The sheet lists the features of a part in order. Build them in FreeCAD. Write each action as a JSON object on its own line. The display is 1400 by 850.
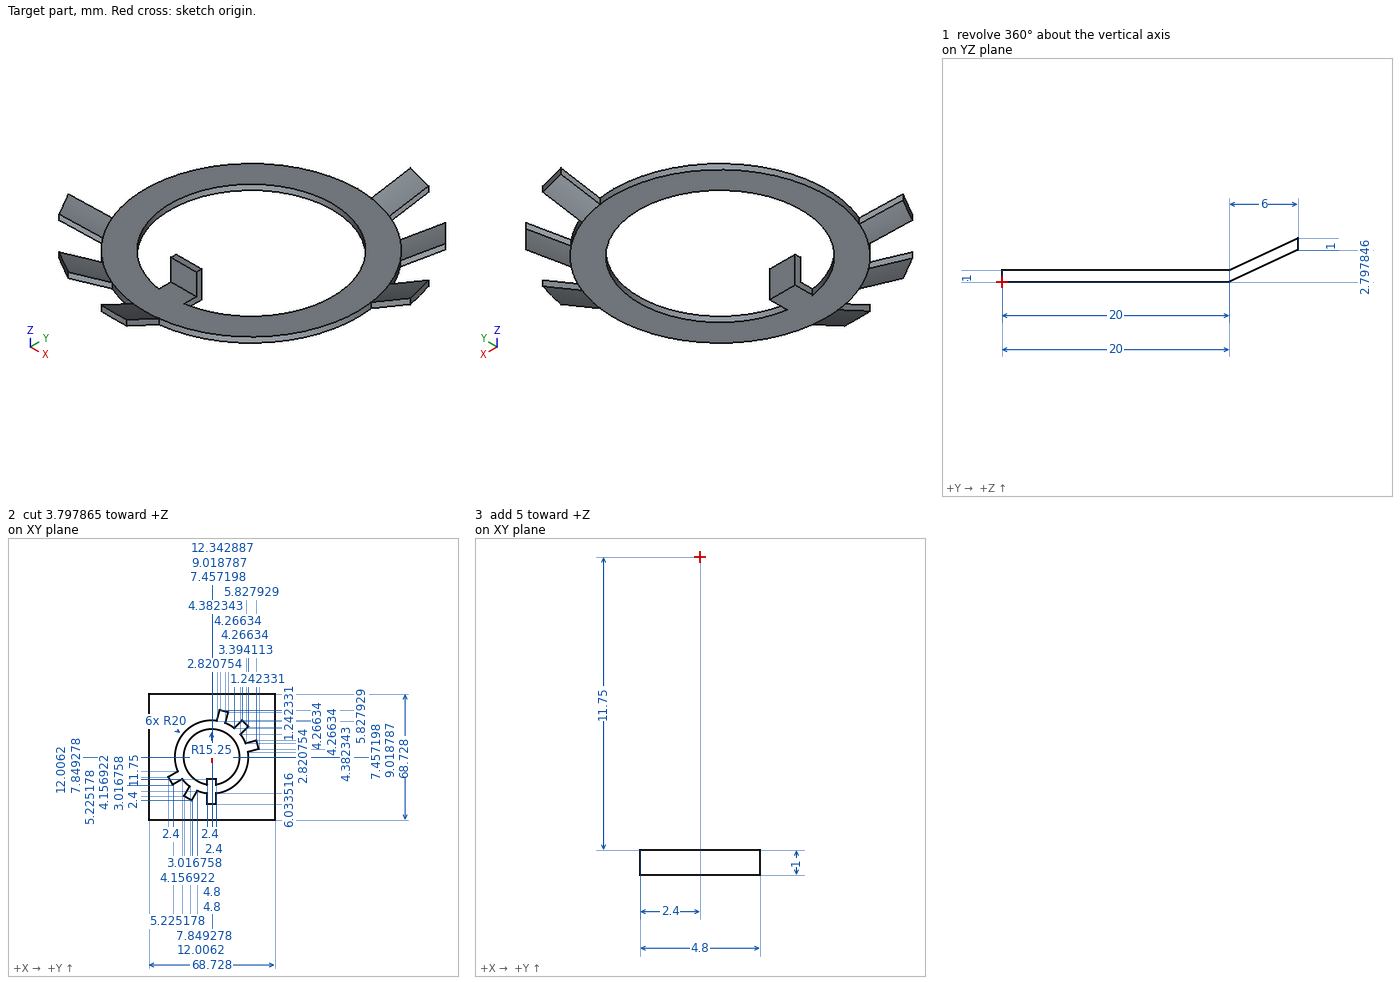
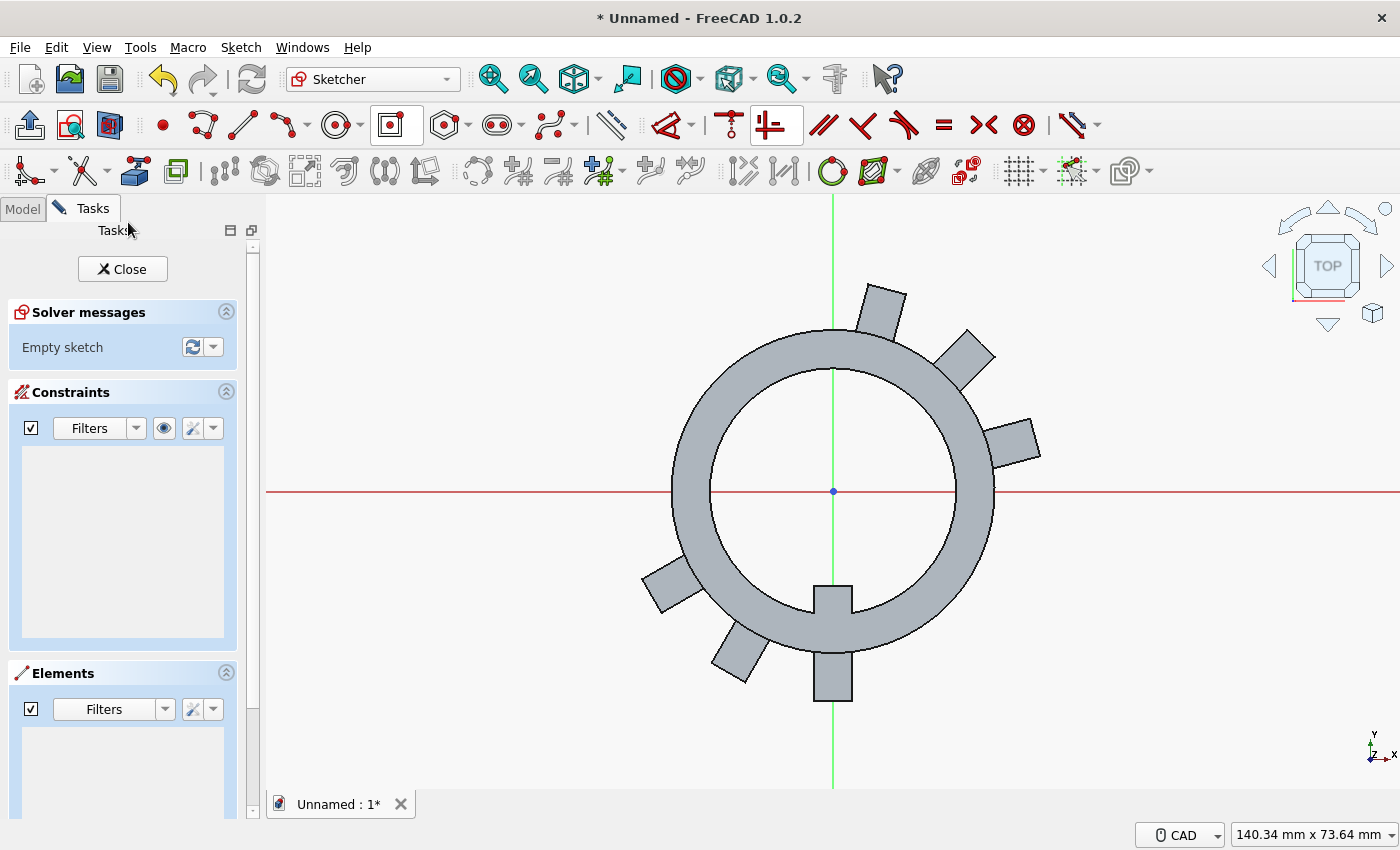
{"action": "left_click", "coordinate": [110, 126]}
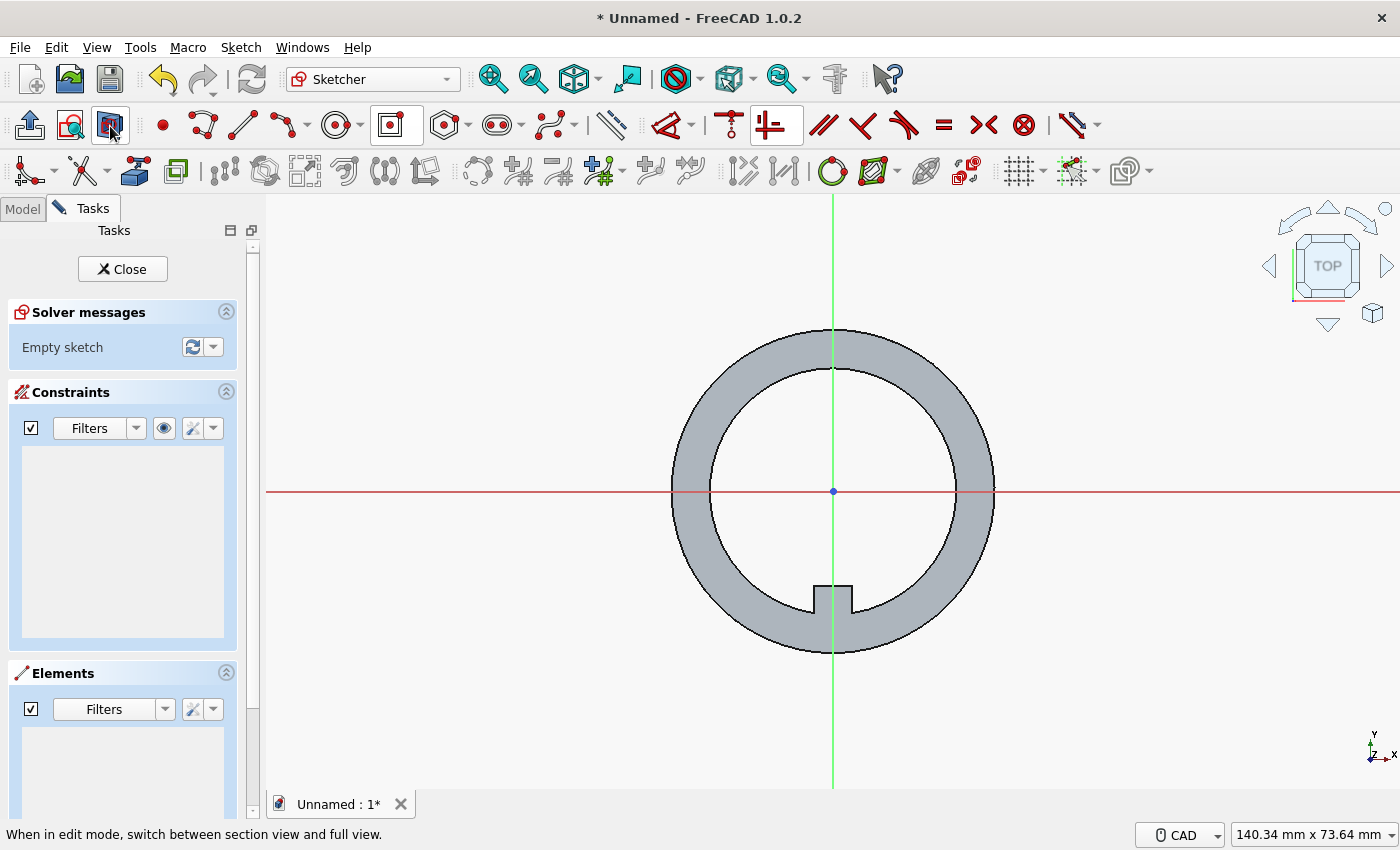
{"action": "scroll", "coordinate": [837, 597], "scroll_direction": "up", "scroll_amount": 14}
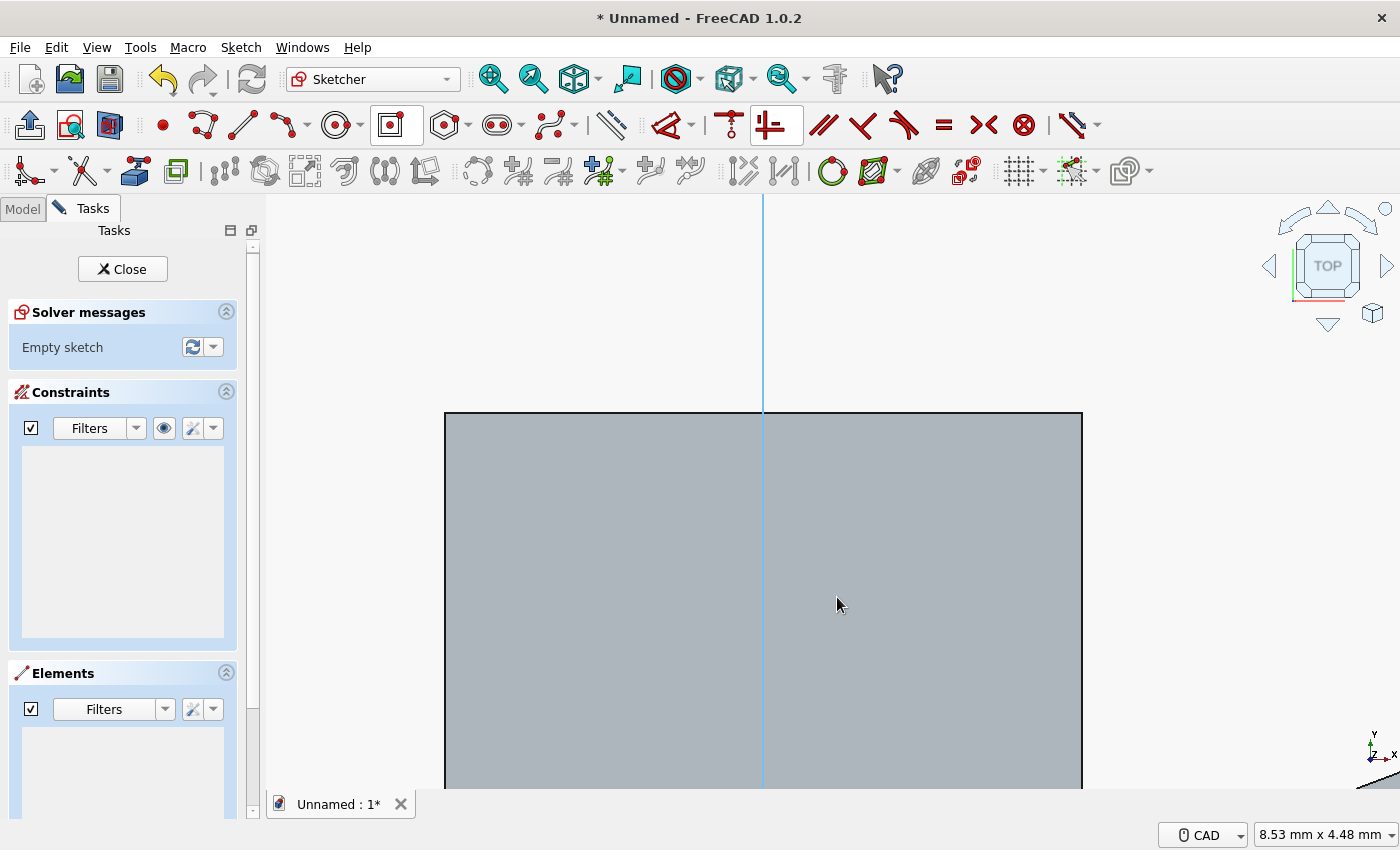
{"action": "left_click", "coordinate": [418, 126]}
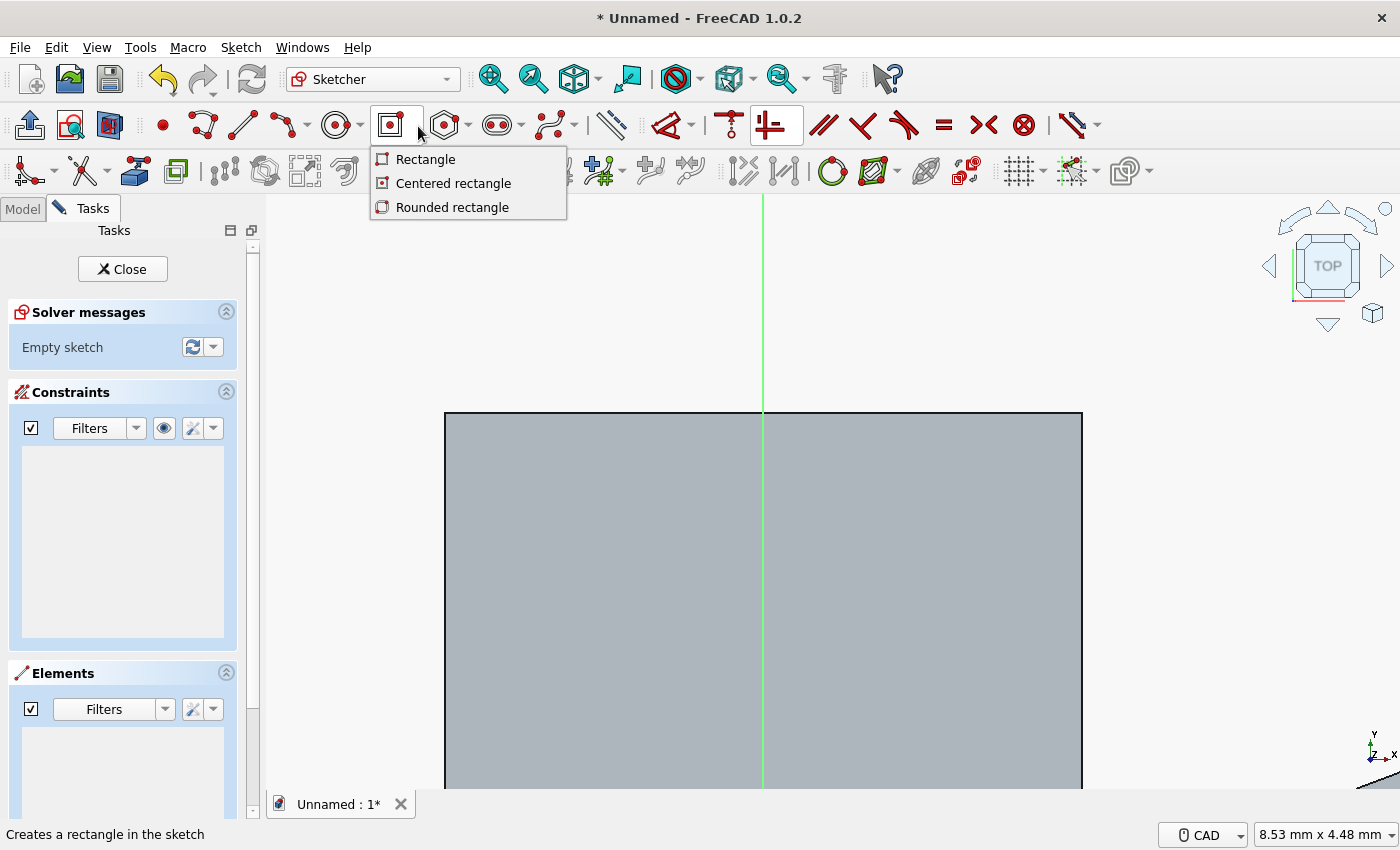
{"action": "left_click", "coordinate": [468, 159]}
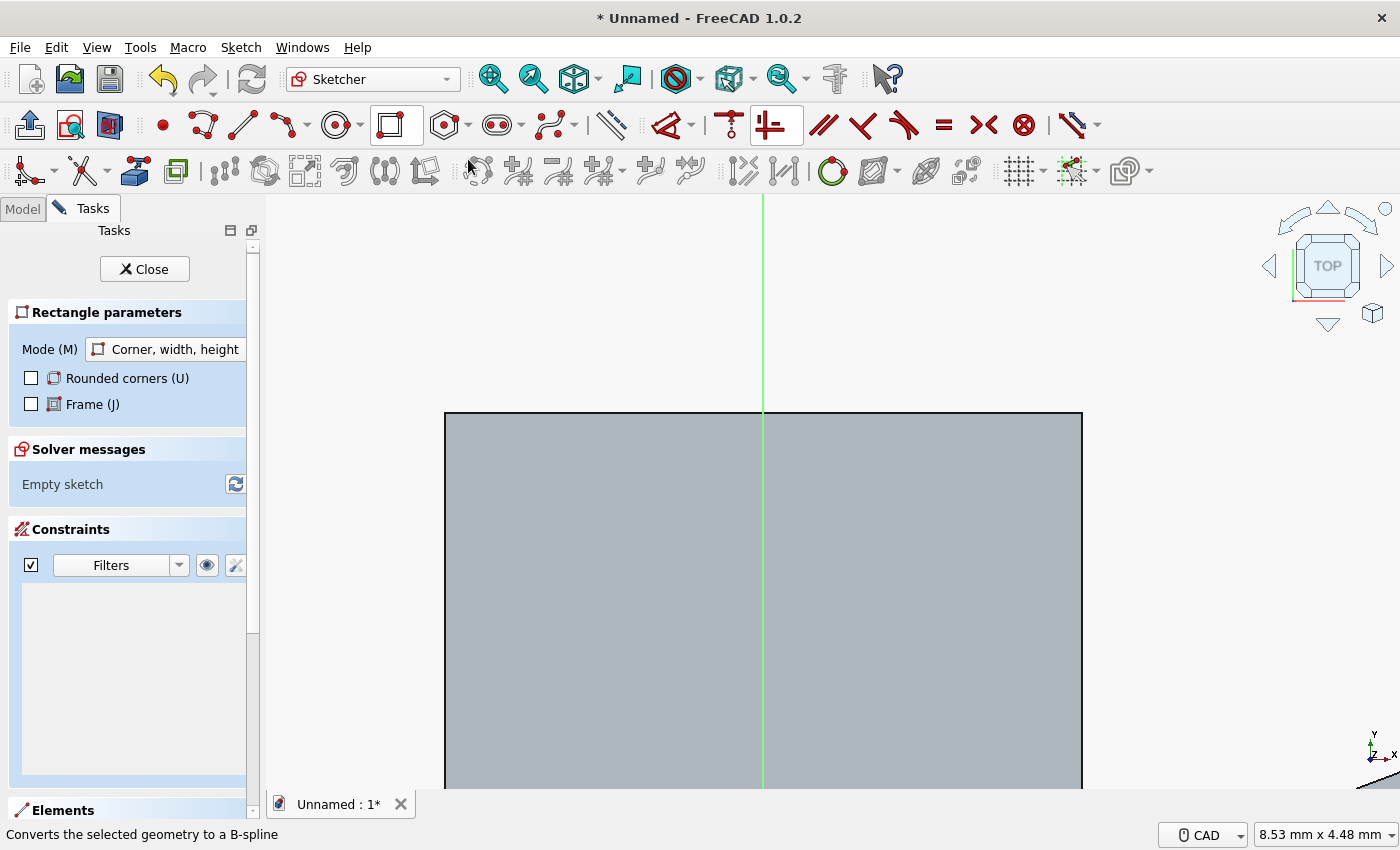
{"action": "left_click", "coordinate": [445, 413]}
{"action": "mouse_move", "coordinate": [1082, 546]}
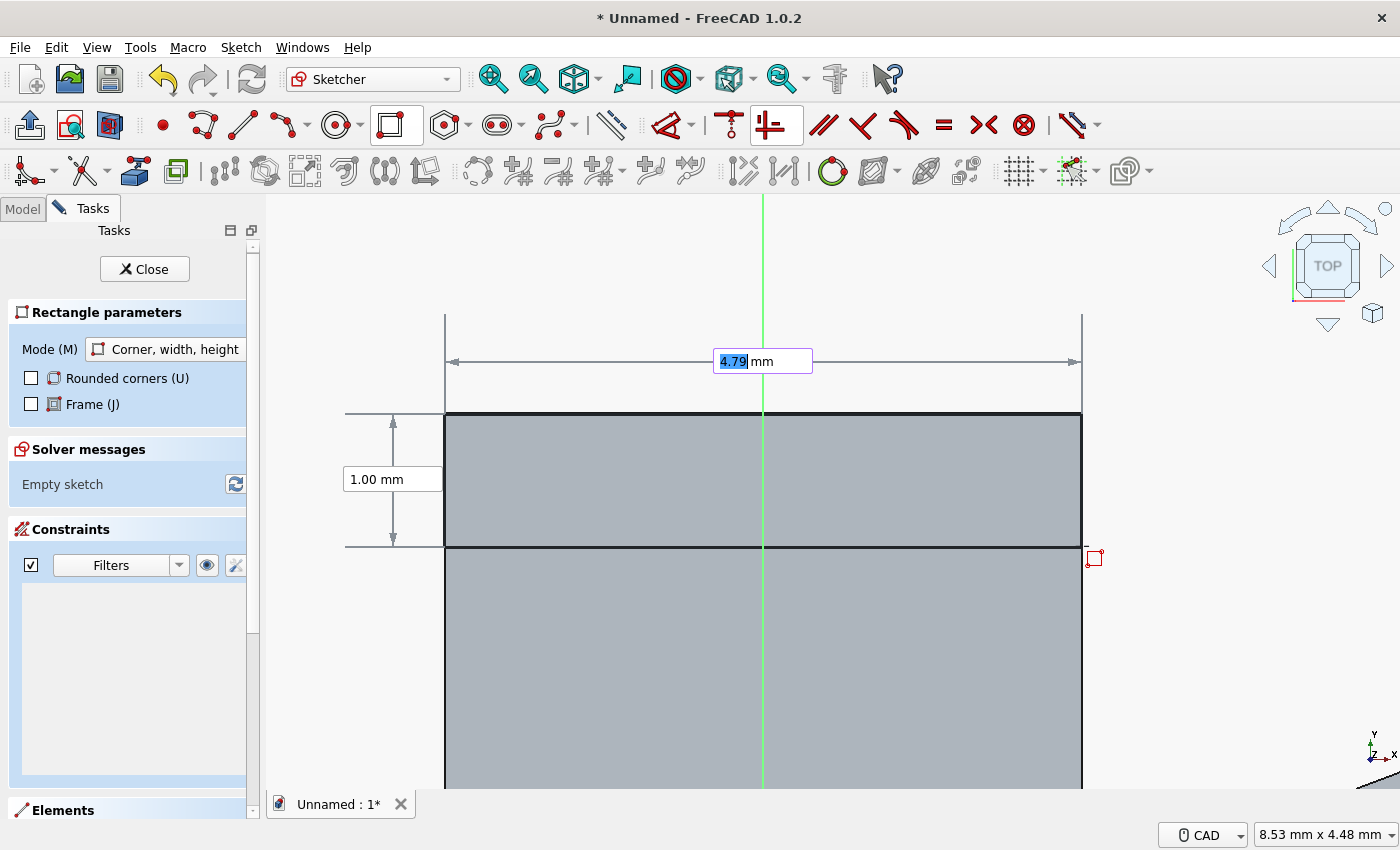
{"action": "type", "text": "4.8"}
{"action": "key", "text": "Tab"}
{"action": "type", "text": "1"}
{"action": "key", "text": "Return"}
{"action": "key", "text": "Escape"}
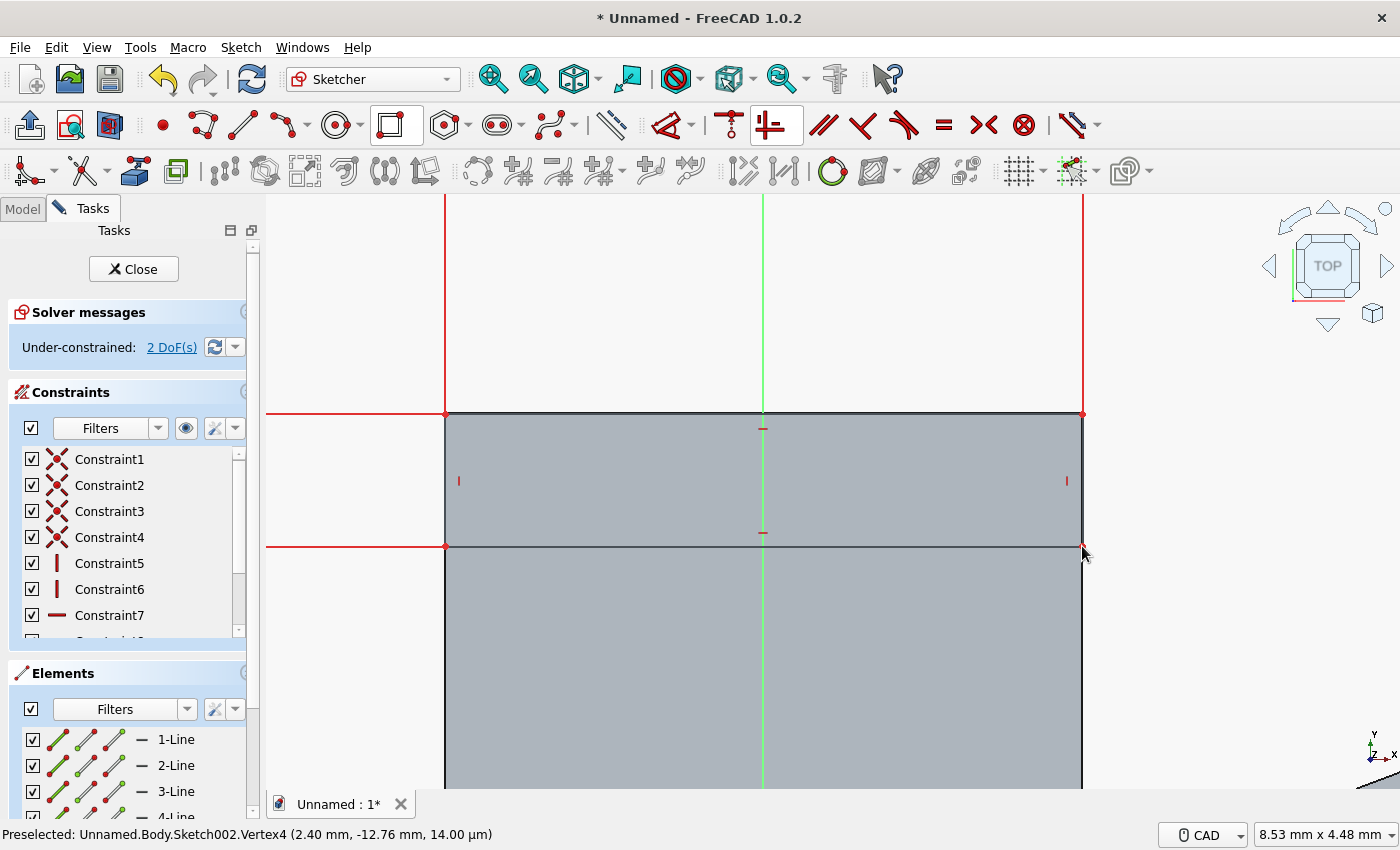
{"action": "left_click", "coordinate": [666, 126]}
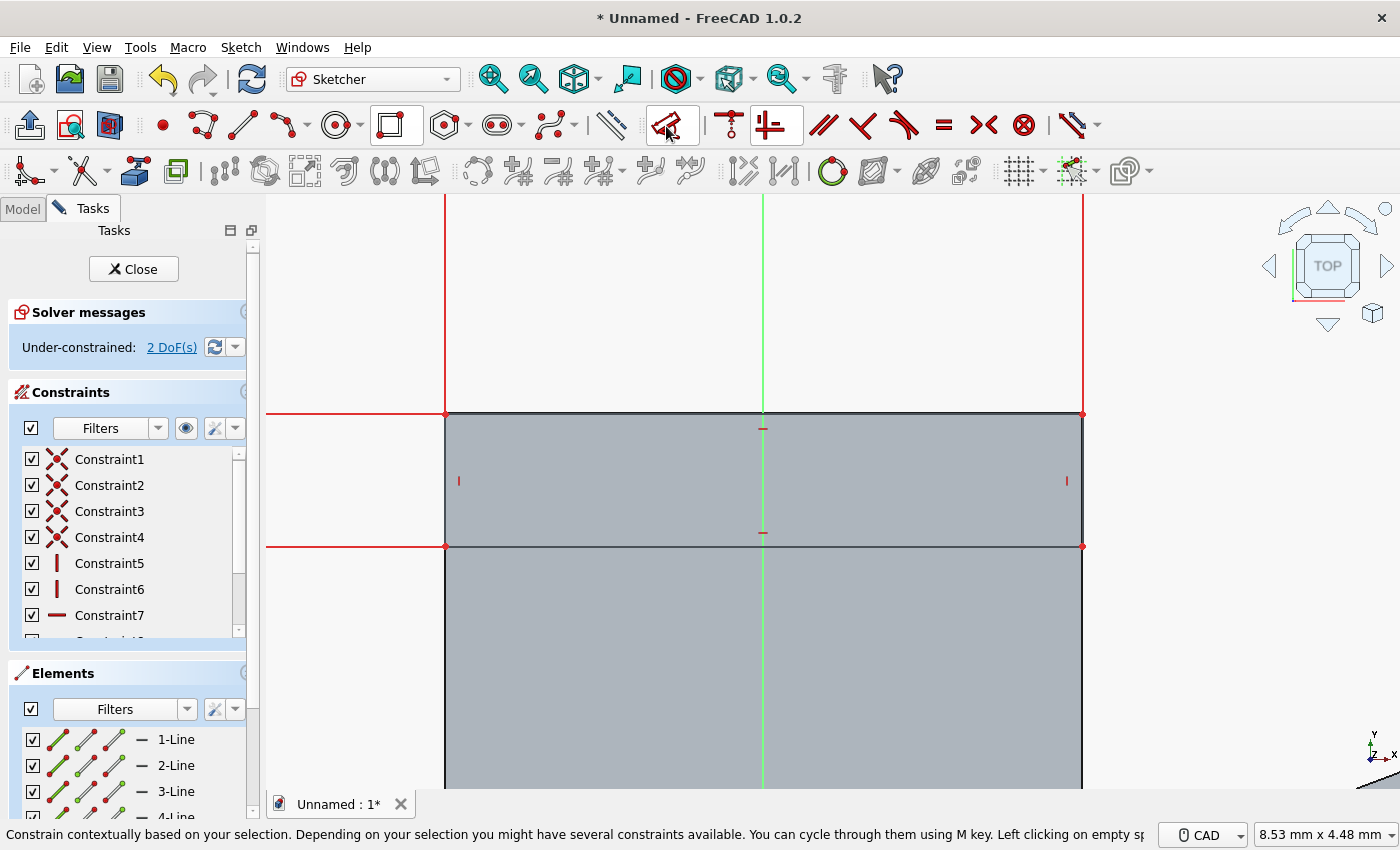
{"action": "left_click", "coordinate": [445, 414]}
{"action": "left_click", "coordinate": [604, 448]}